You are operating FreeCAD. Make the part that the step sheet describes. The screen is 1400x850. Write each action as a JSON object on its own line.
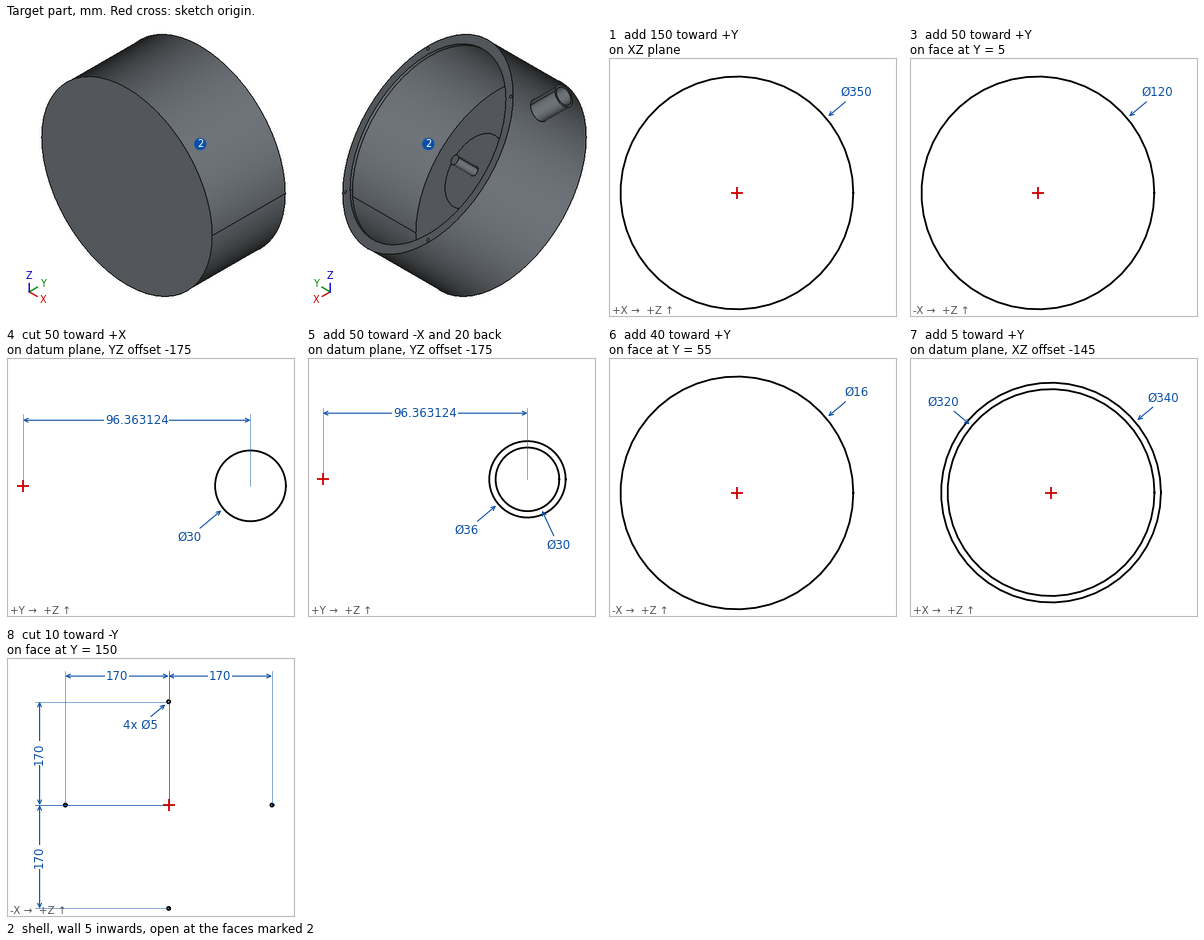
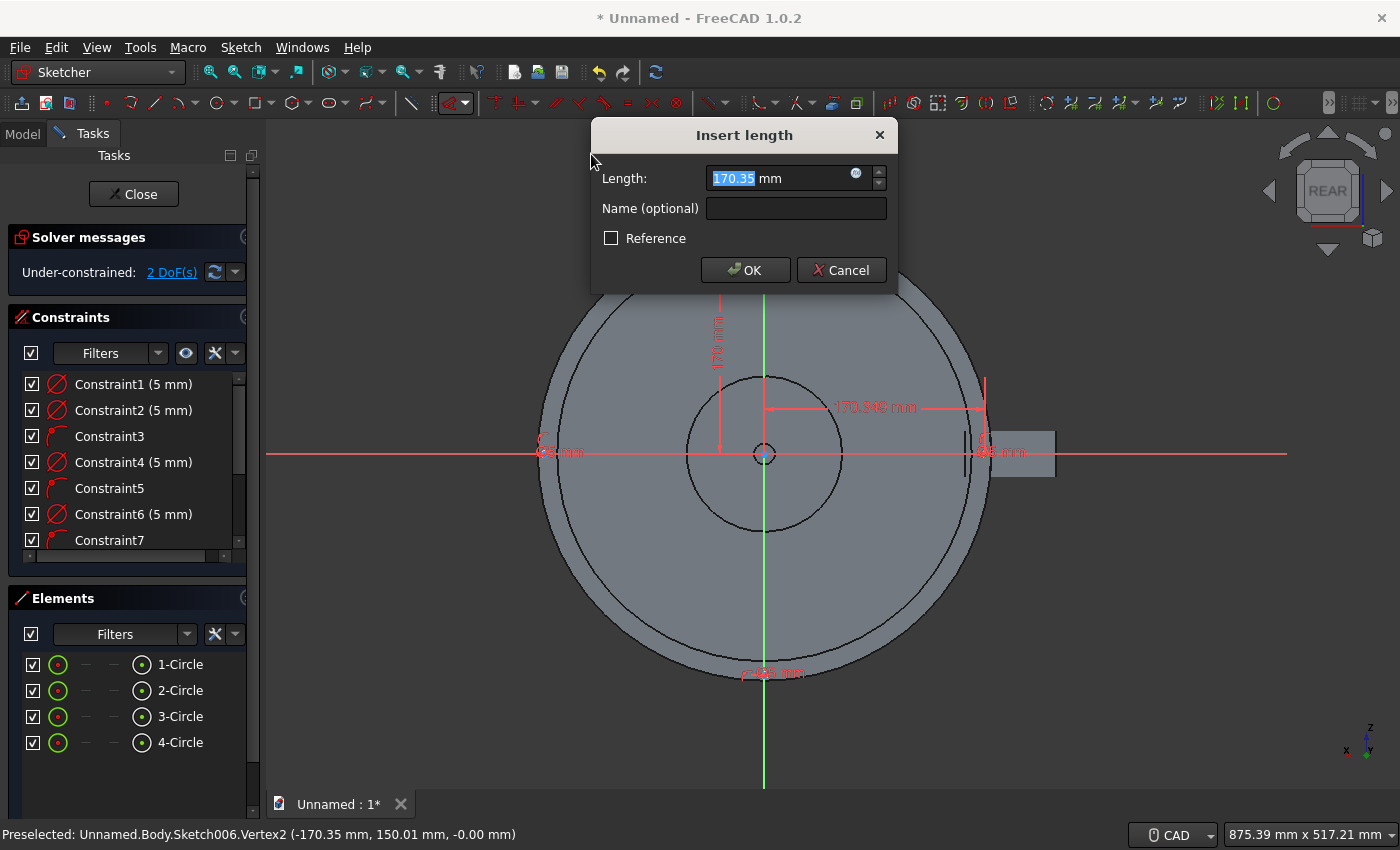
{"action": "type", "text": "170"}
{"action": "key", "text": "Return"}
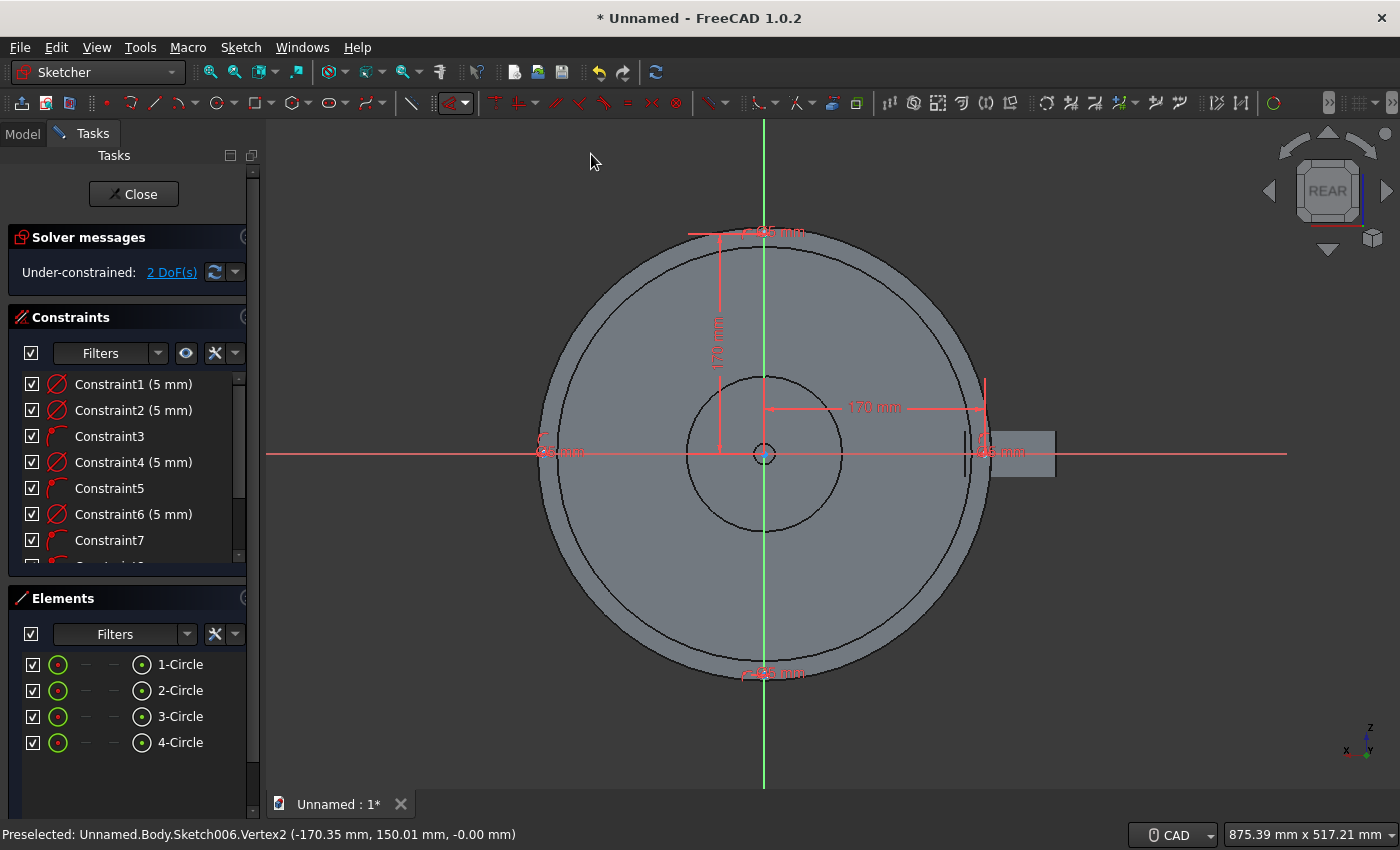
{"action": "left_click", "coordinate": [764, 675]}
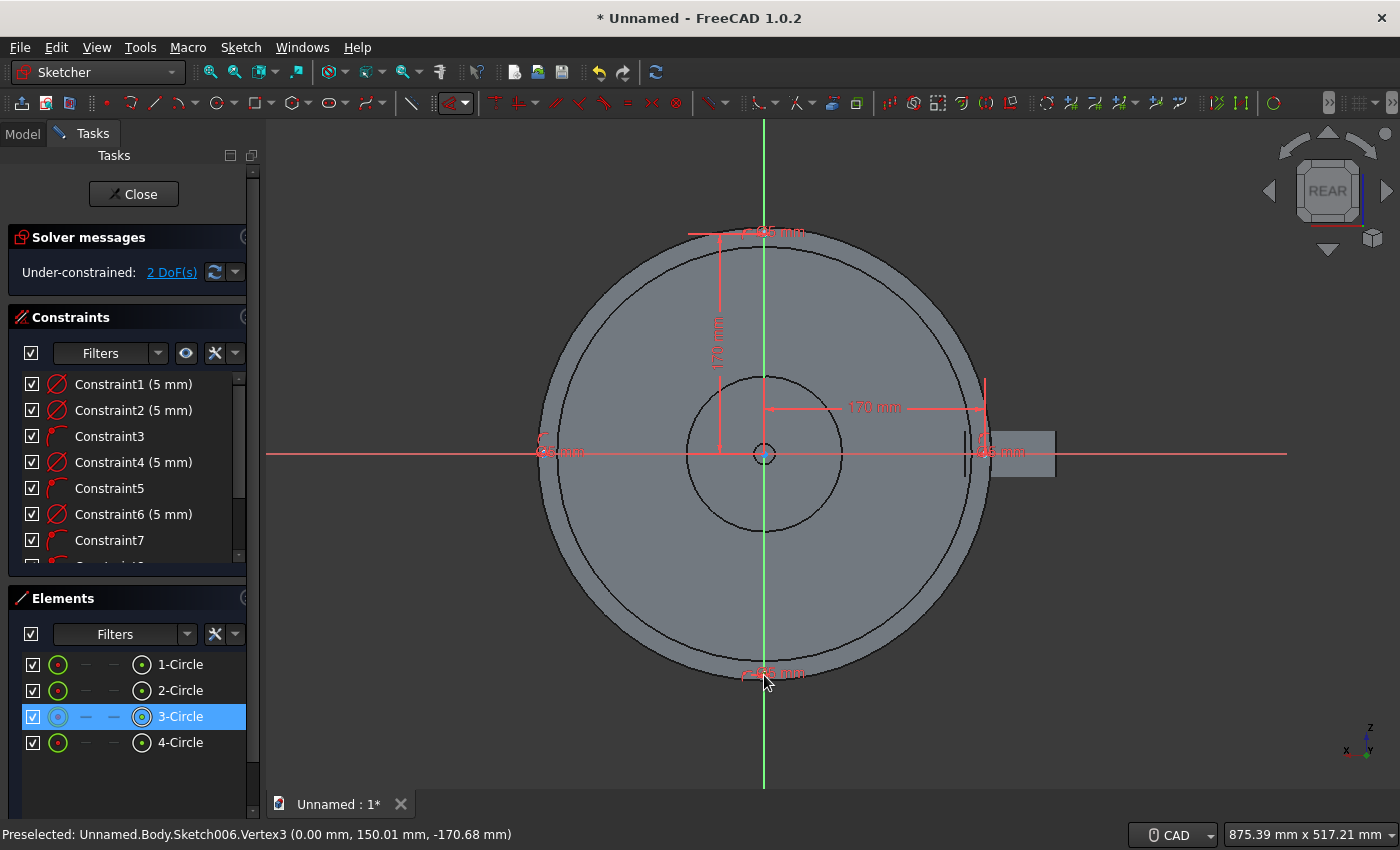
{"action": "left_click", "coordinate": [468, 104]}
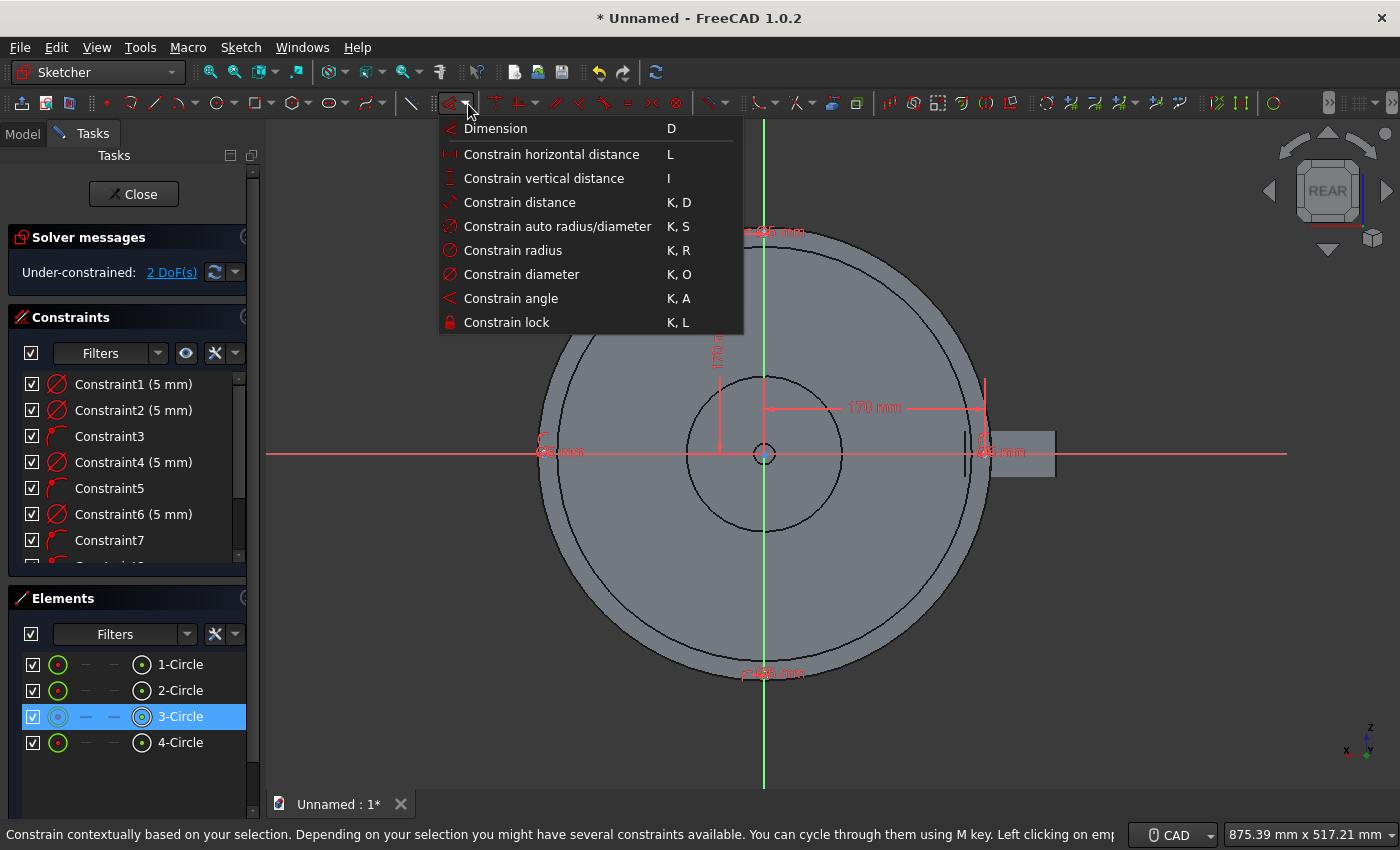
{"action": "left_click", "coordinate": [591, 178]}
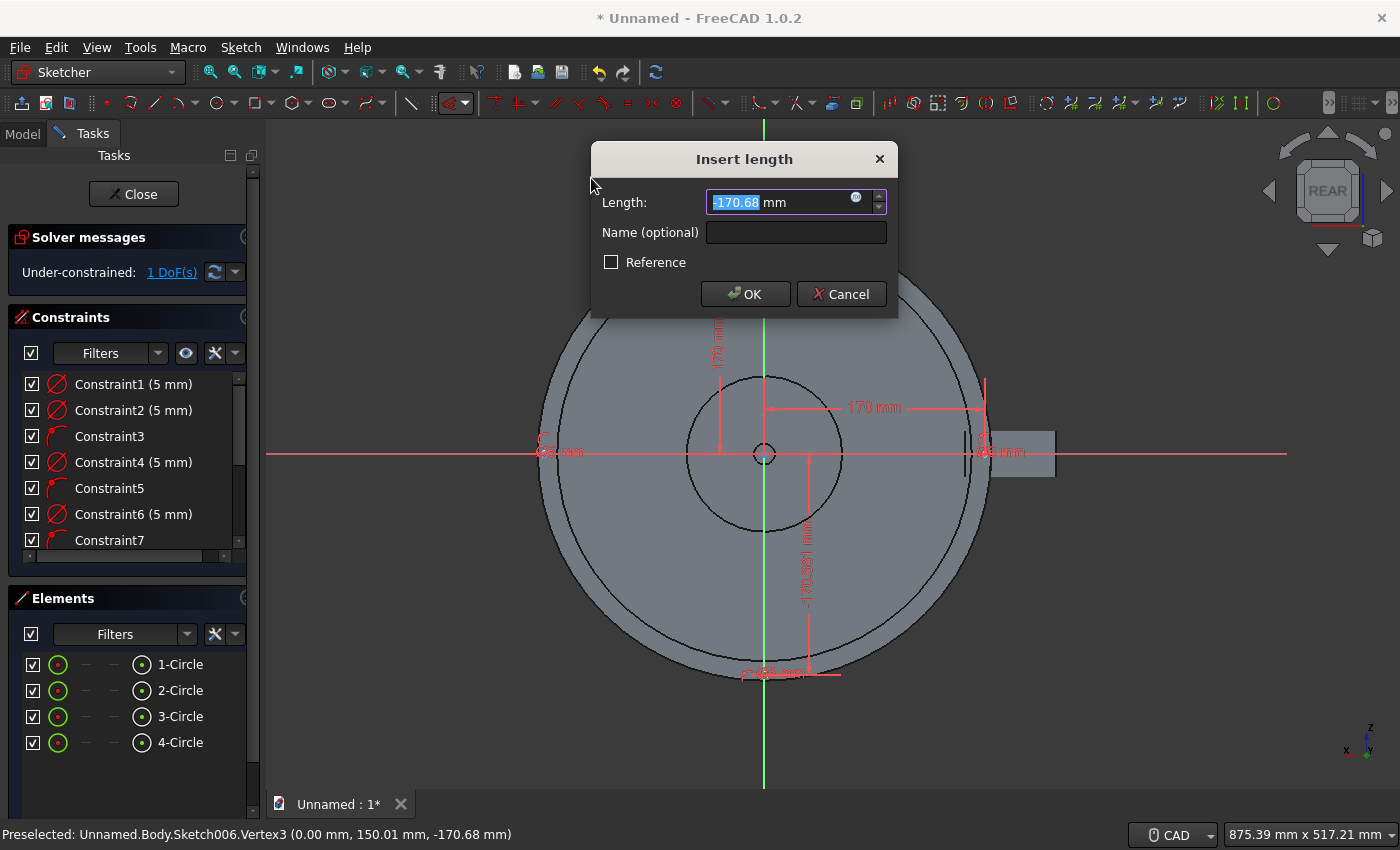
{"action": "type", "text": "-170"}
{"action": "key", "text": "Return"}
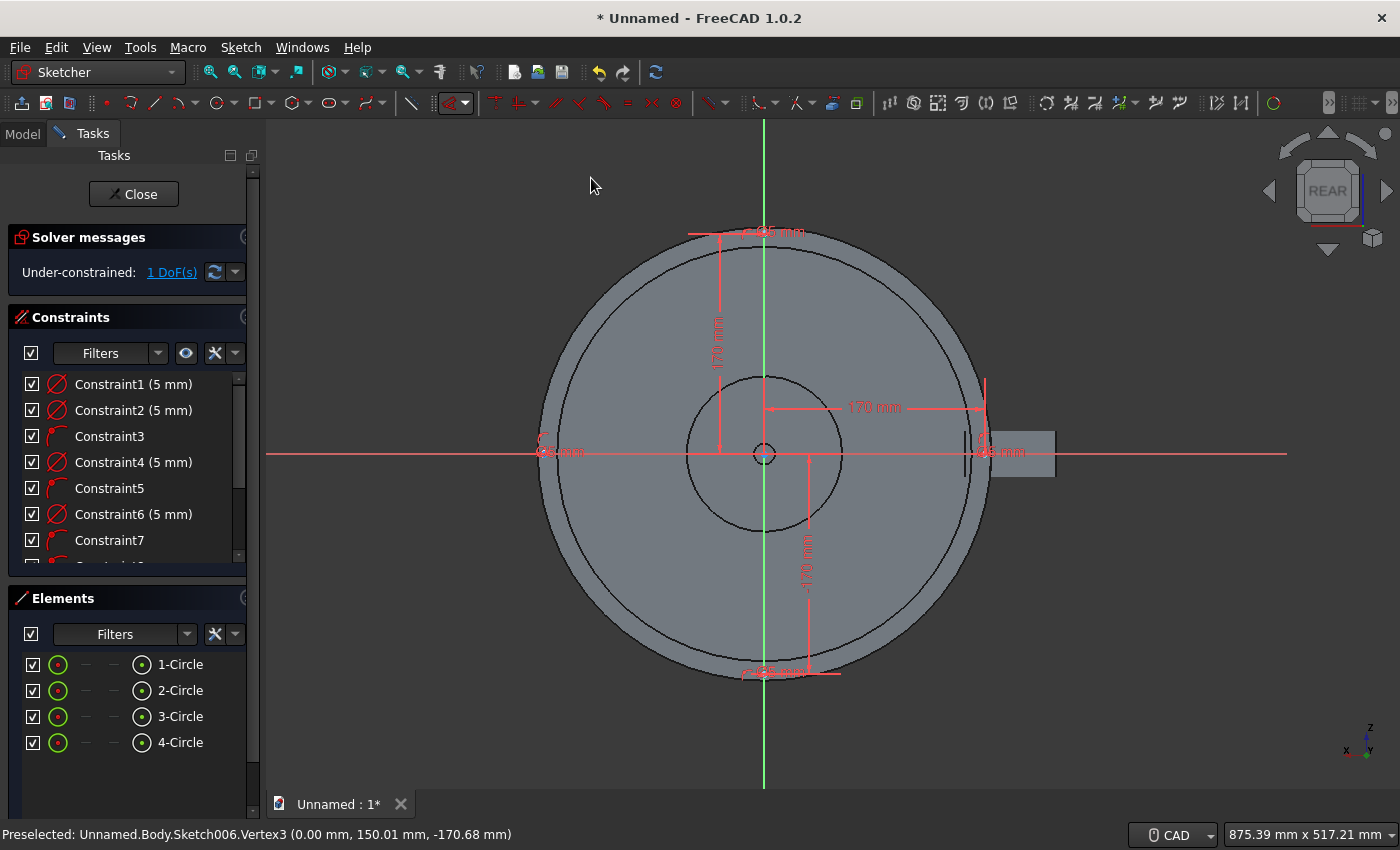
{"action": "left_click", "coordinate": [544, 454]}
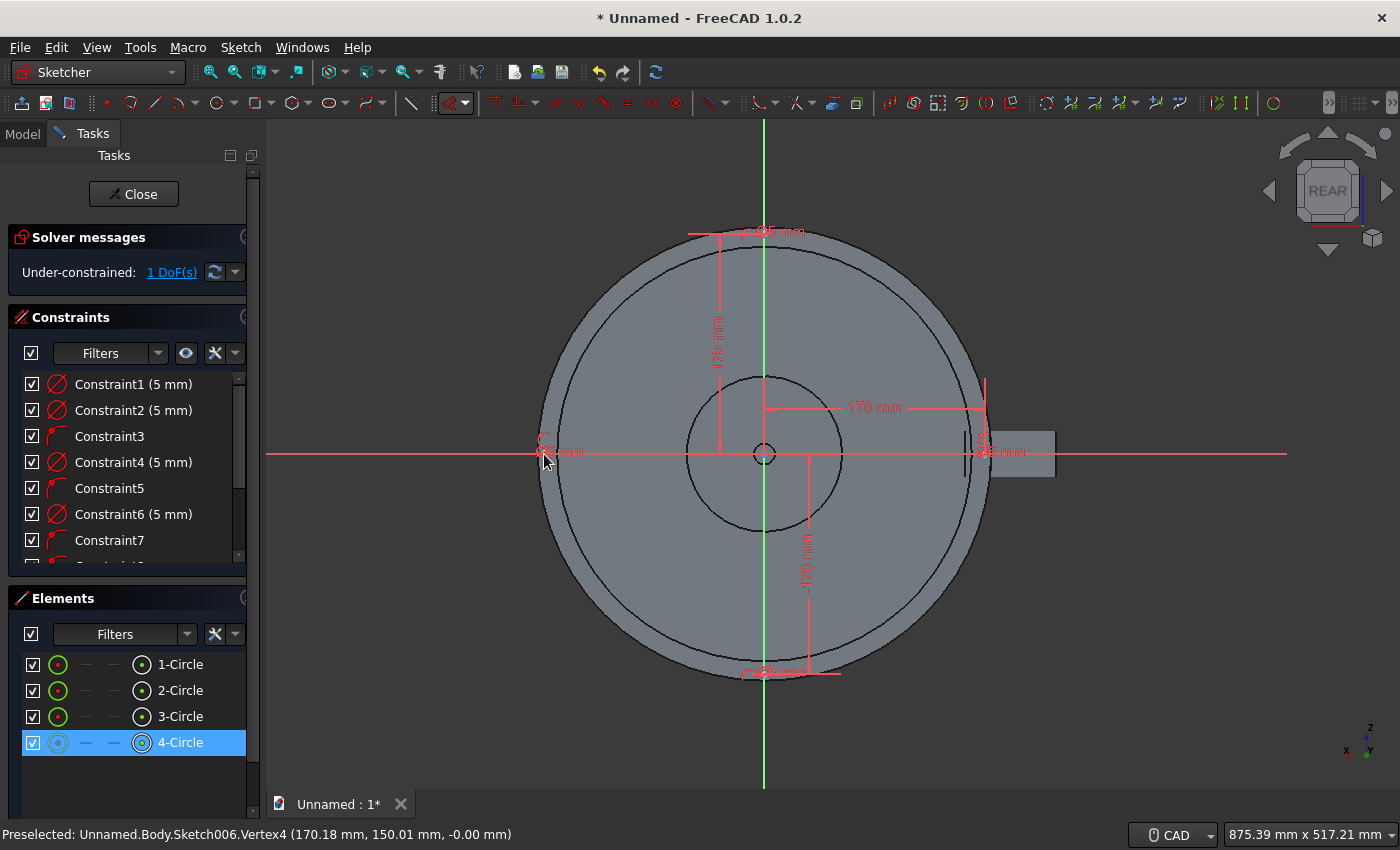
{"action": "key", "text": "l"}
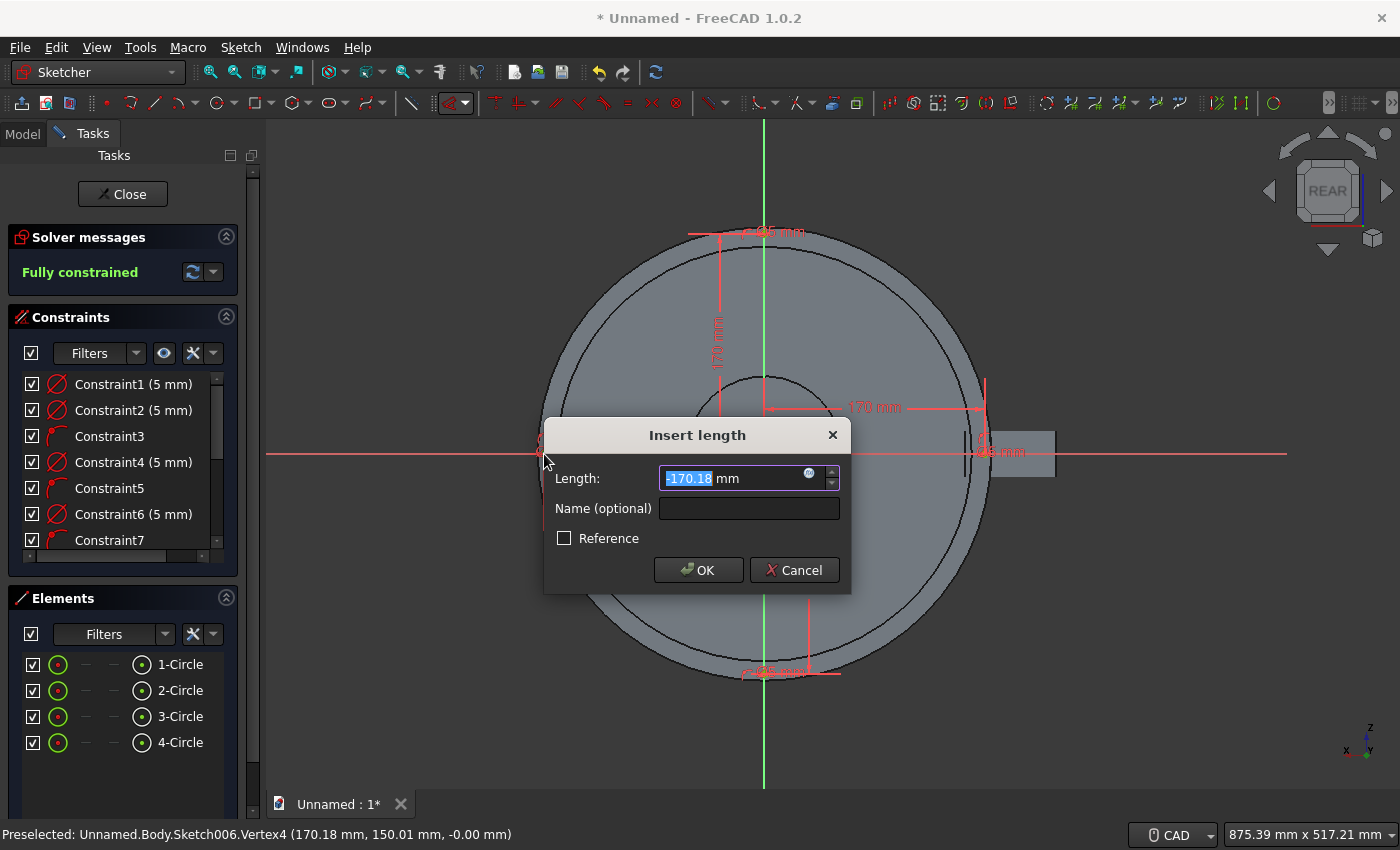
{"action": "type", "text": "-170"}
{"action": "key", "text": "Return"}